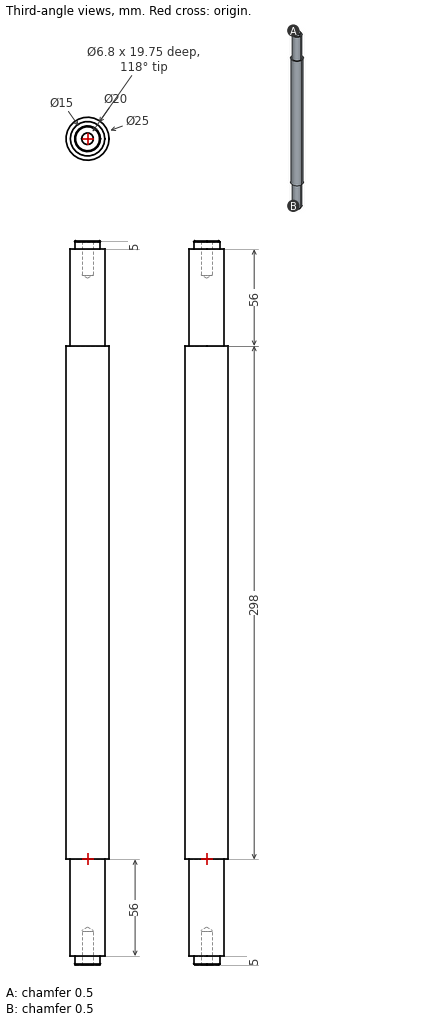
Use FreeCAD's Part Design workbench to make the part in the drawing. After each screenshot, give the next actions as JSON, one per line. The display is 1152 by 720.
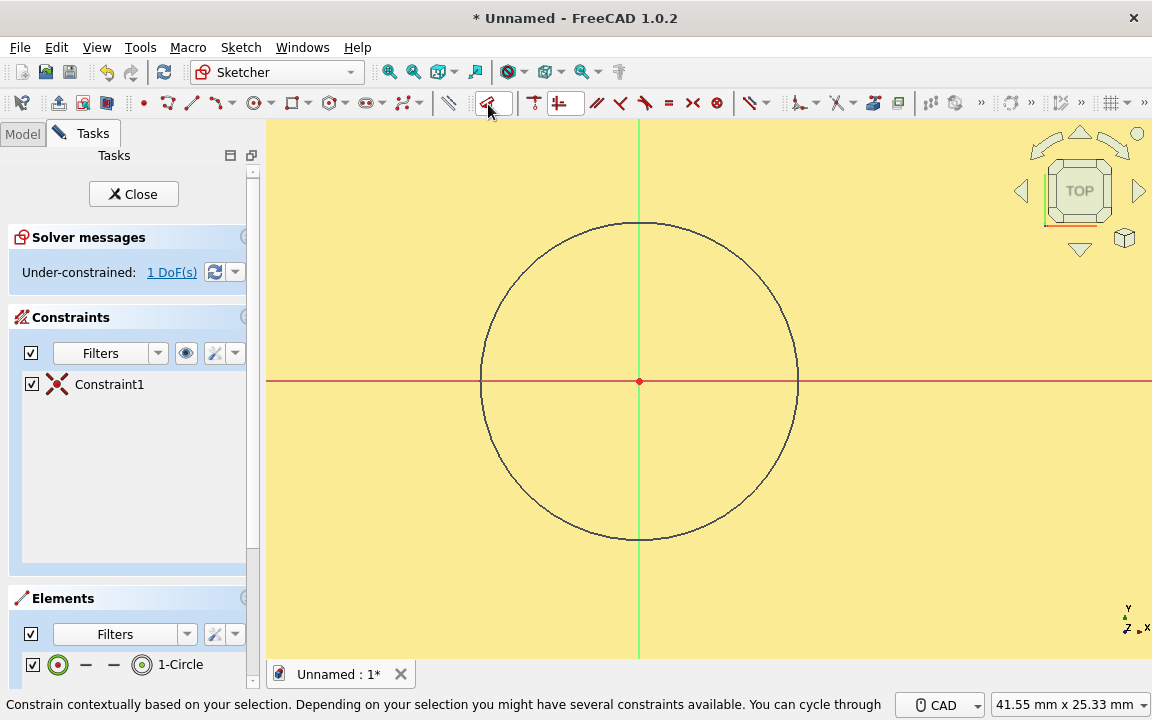
{"action": "left_click", "coordinate": [751, 268]}
{"action": "left_click", "coordinate": [773, 245]}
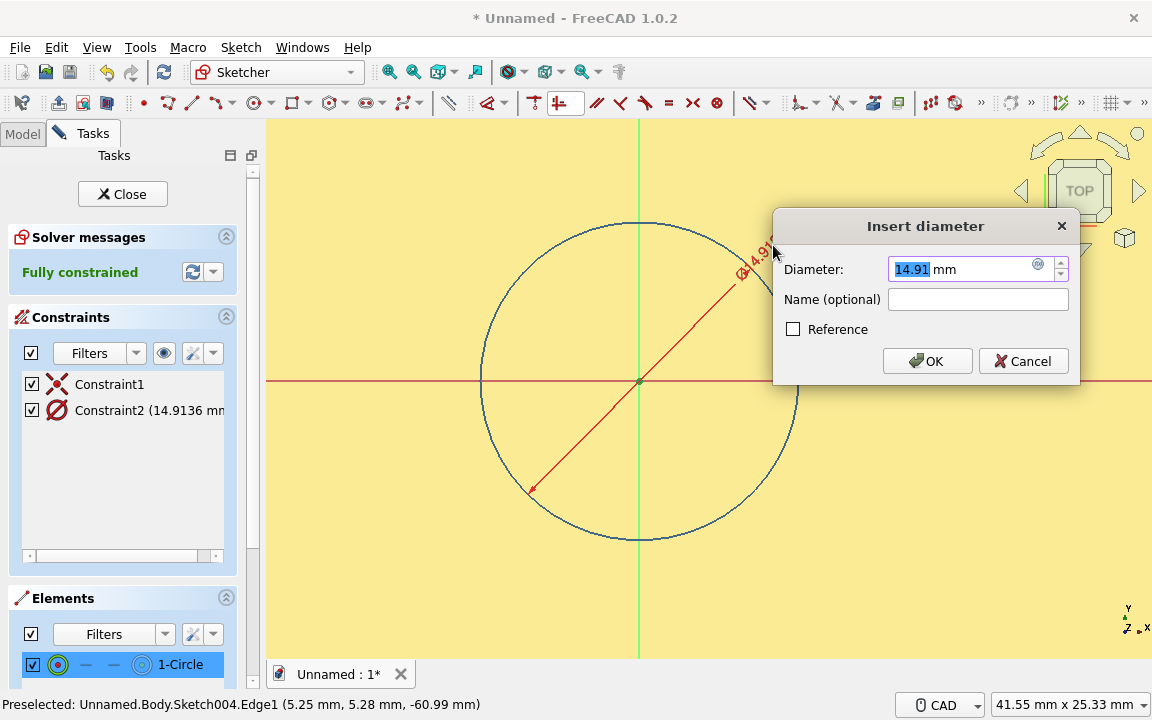
{"action": "type", "text": "15"}
{"action": "key", "text": "Return"}
{"action": "key", "text": "Escape"}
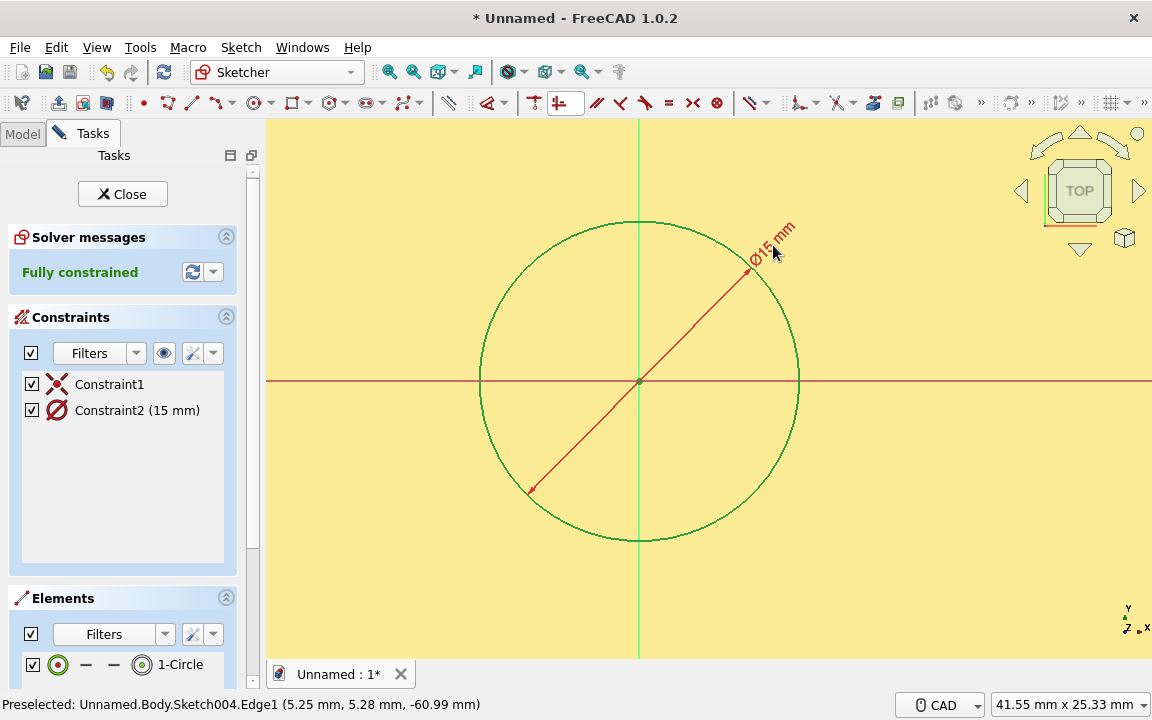
{"action": "left_click", "coordinate": [123, 194]}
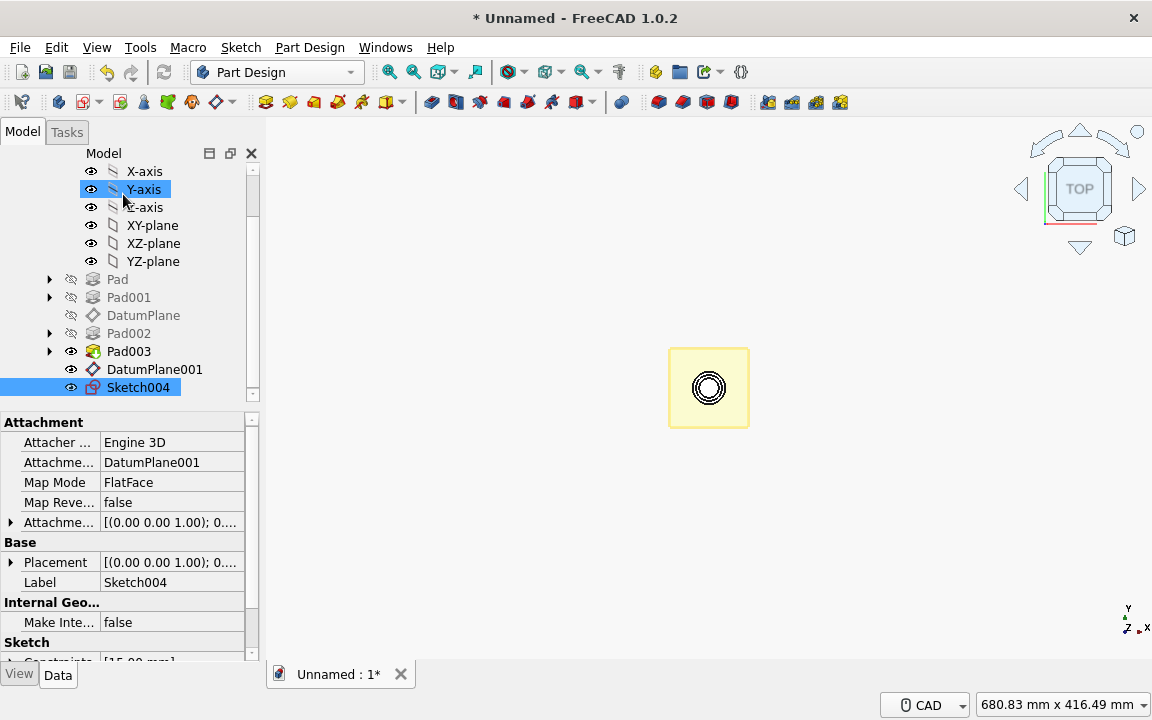
{"action": "left_click", "coordinate": [266, 102]}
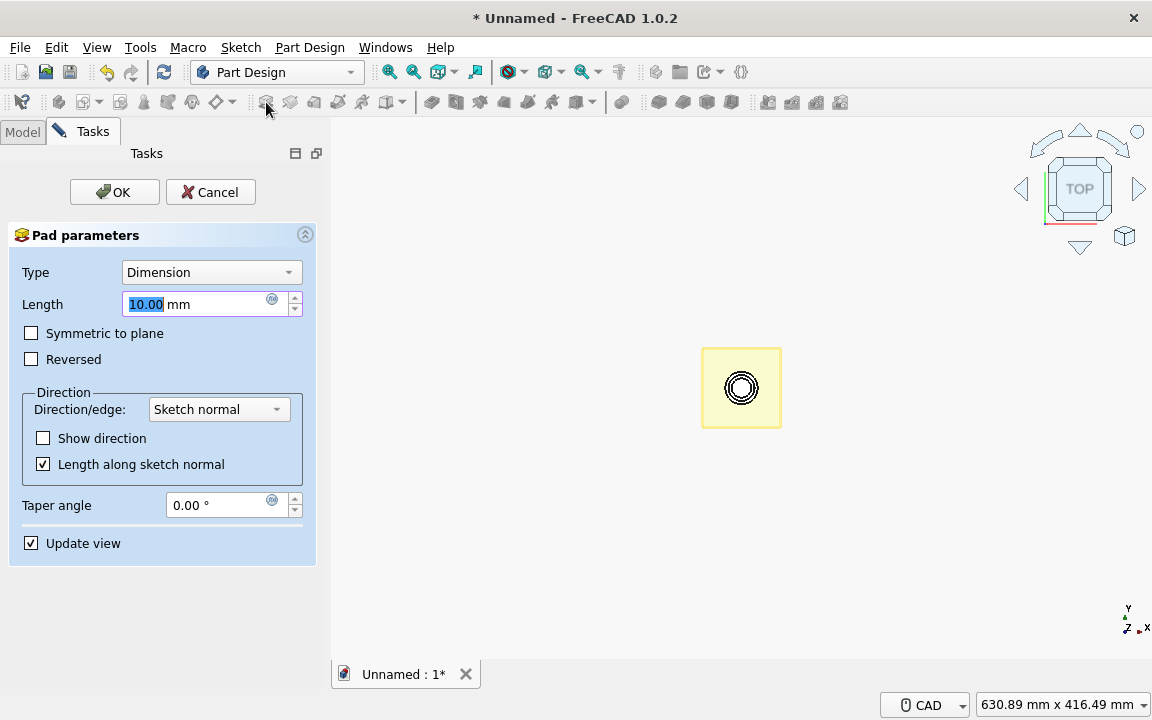
{"action": "type", "text": "5"}
{"action": "key", "text": "Tab"}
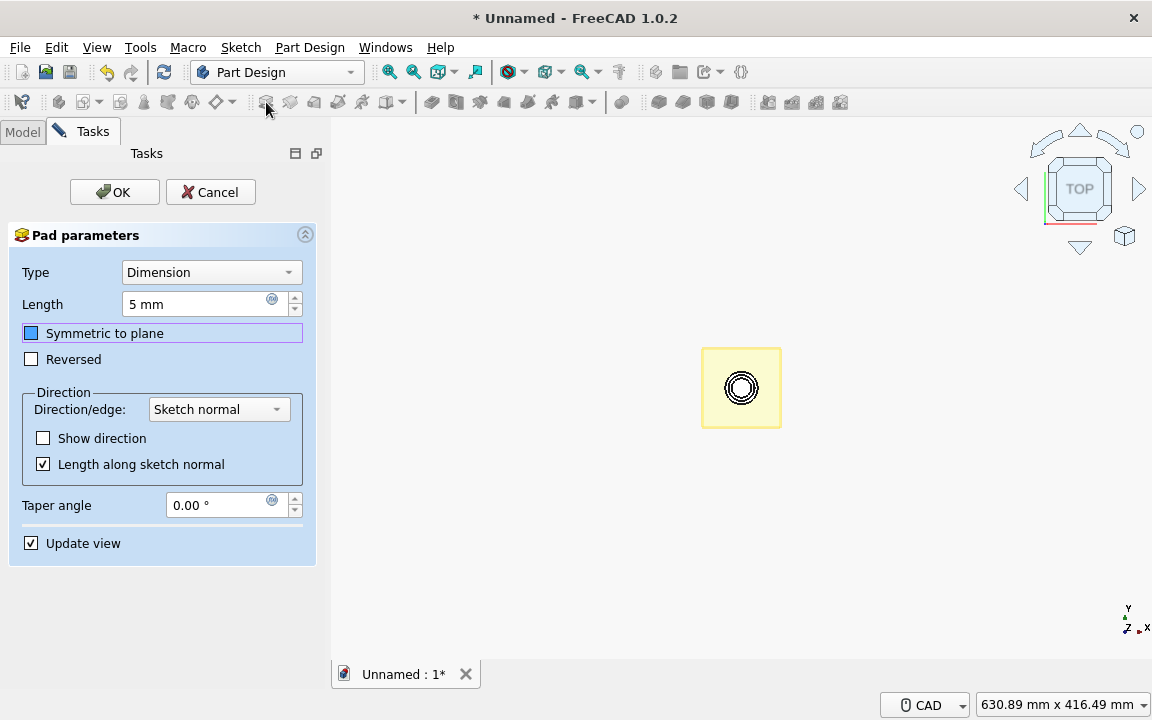
{"action": "left_click", "coordinate": [115, 192]}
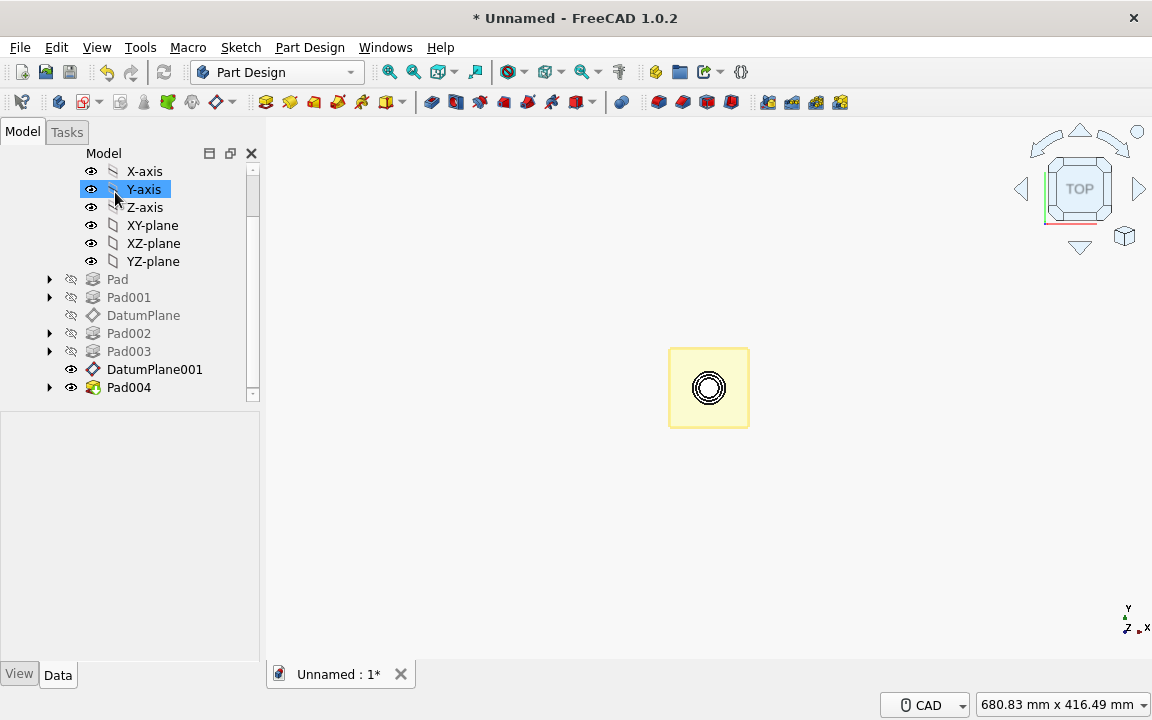
{"action": "left_click", "coordinate": [116, 369]}
{"action": "key", "text": "space"}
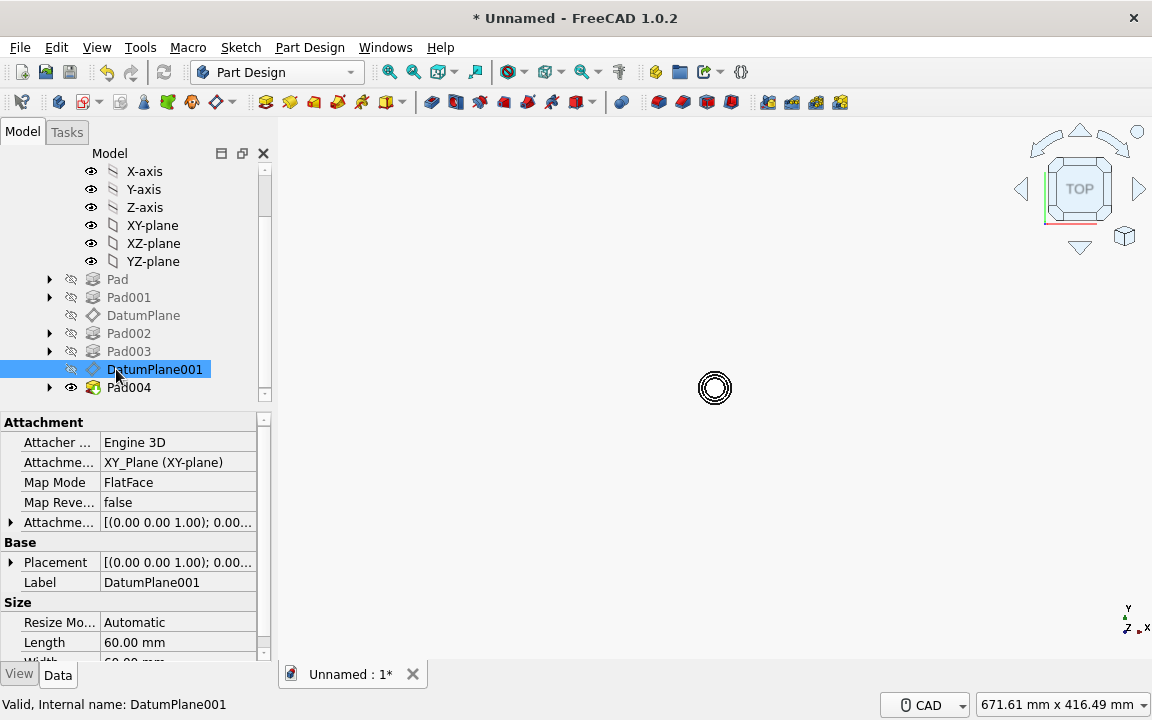
{"action": "left_click", "coordinate": [390, 72]}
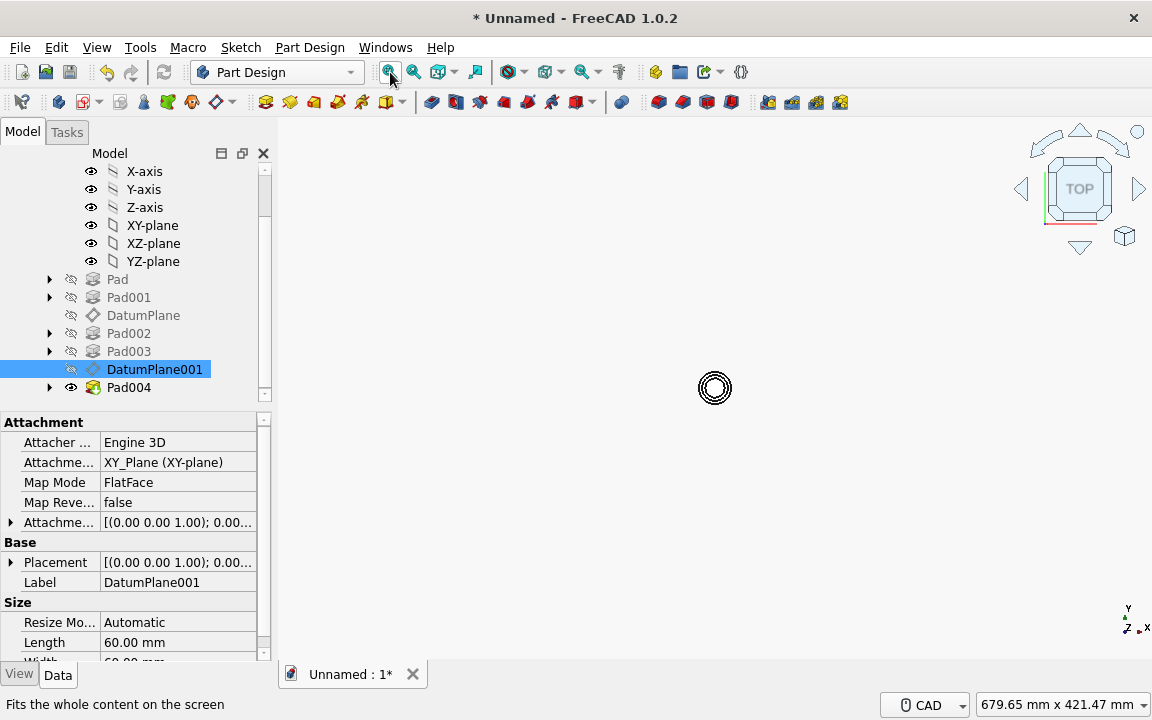
{"action": "key", "text": "5"}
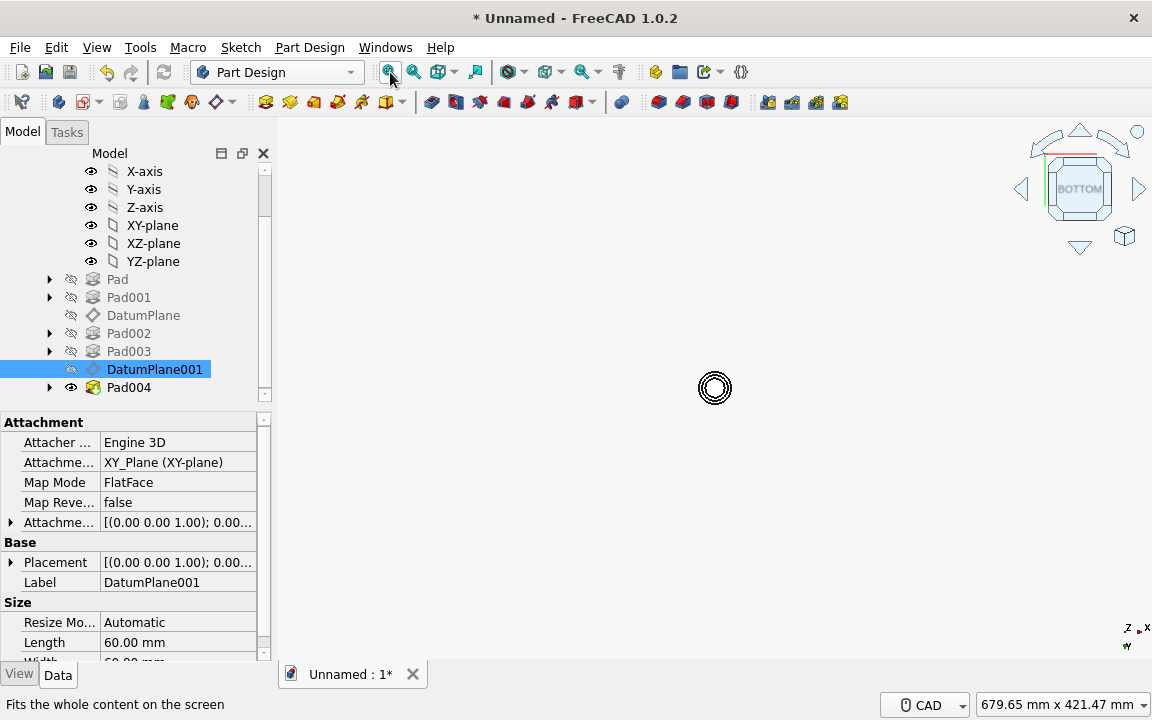
{"action": "left_click", "coordinate": [390, 72]}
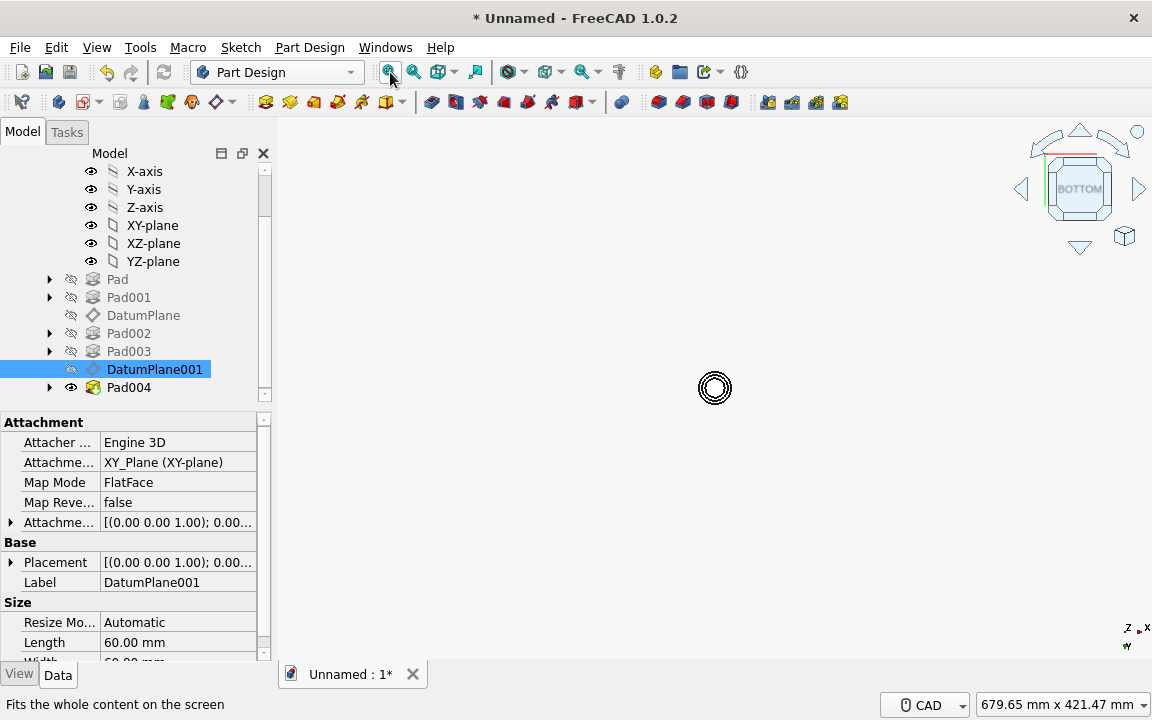
{"action": "left_click", "coordinate": [715, 387]}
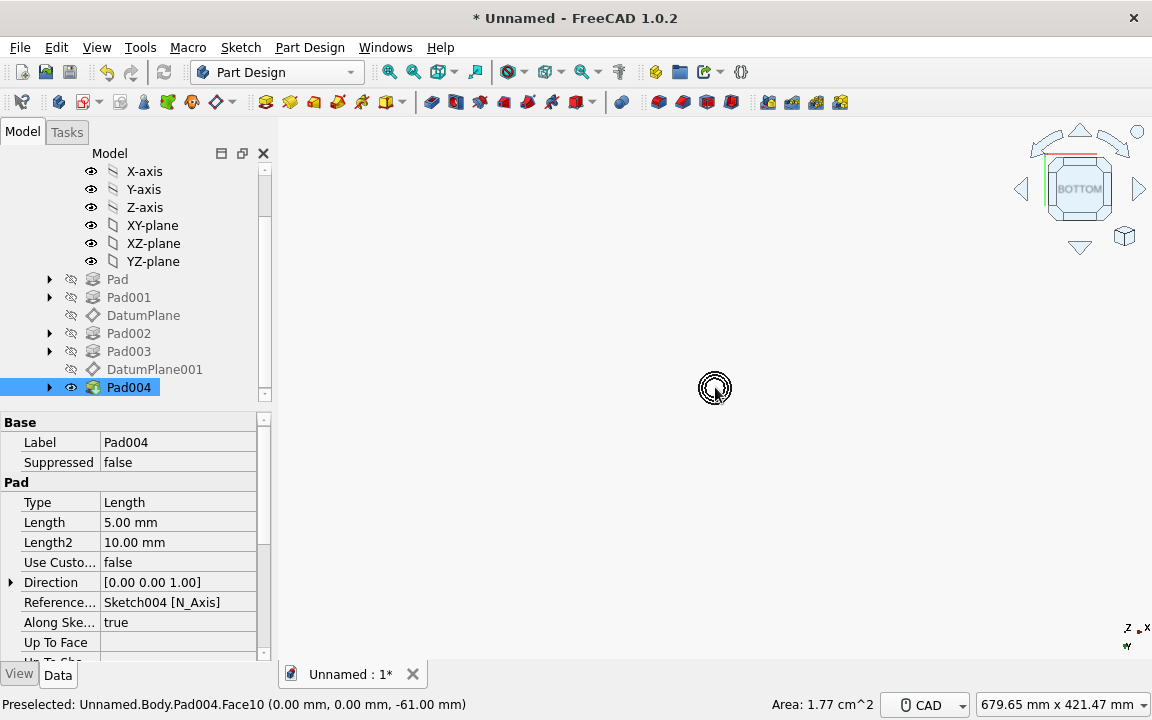
{"action": "left_click", "coordinate": [84, 102]}